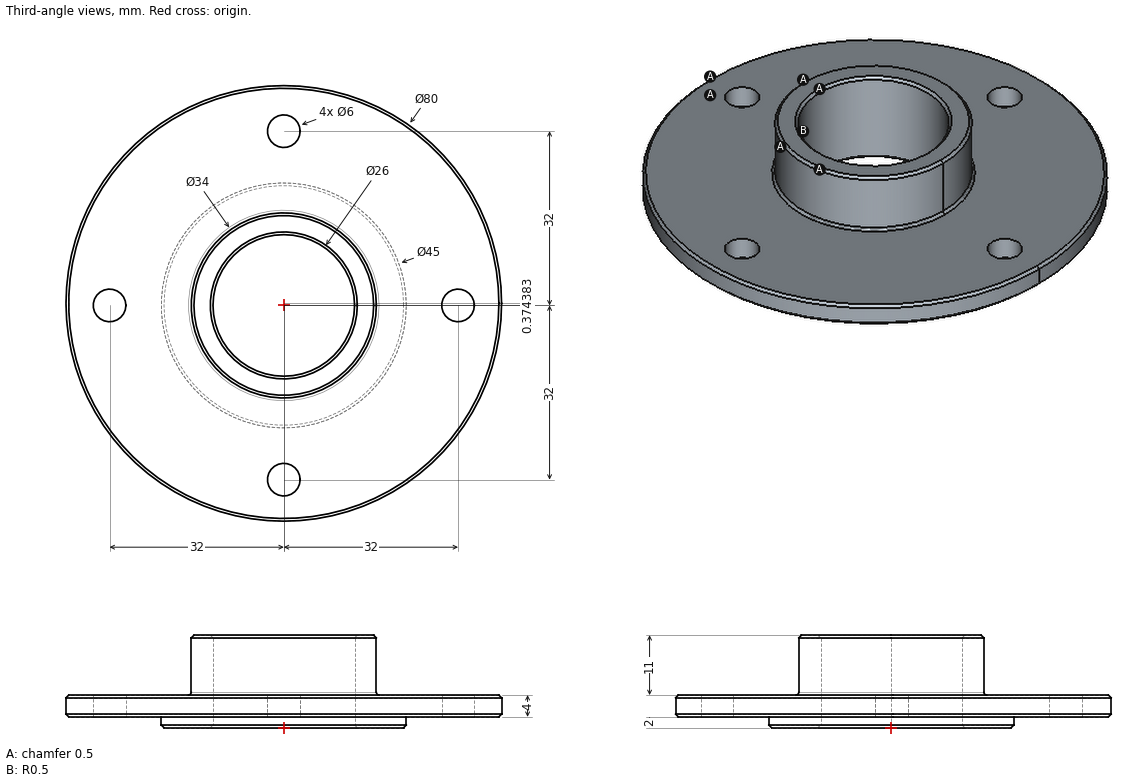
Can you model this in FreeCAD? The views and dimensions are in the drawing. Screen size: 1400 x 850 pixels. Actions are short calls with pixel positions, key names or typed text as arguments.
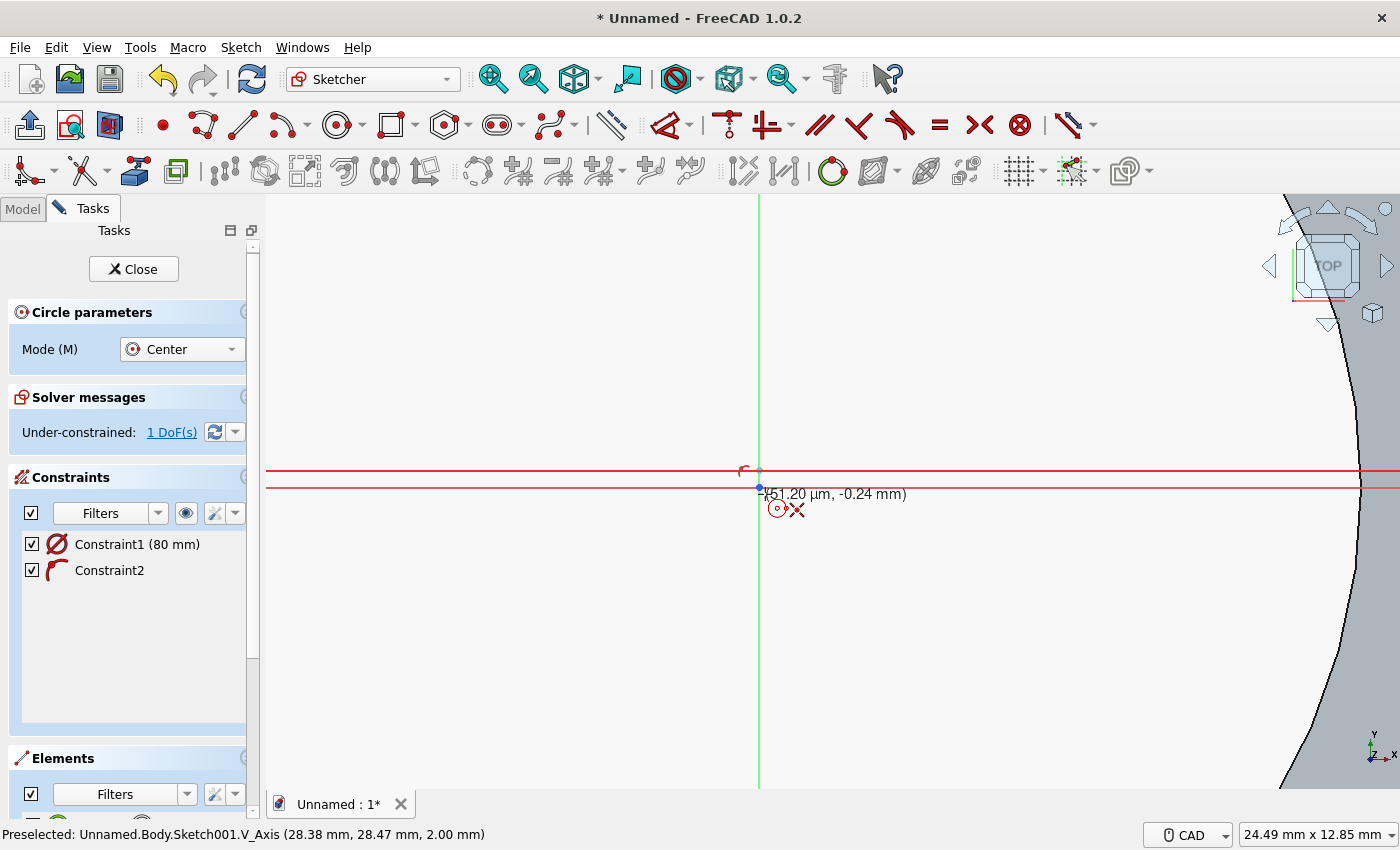
click(759, 488)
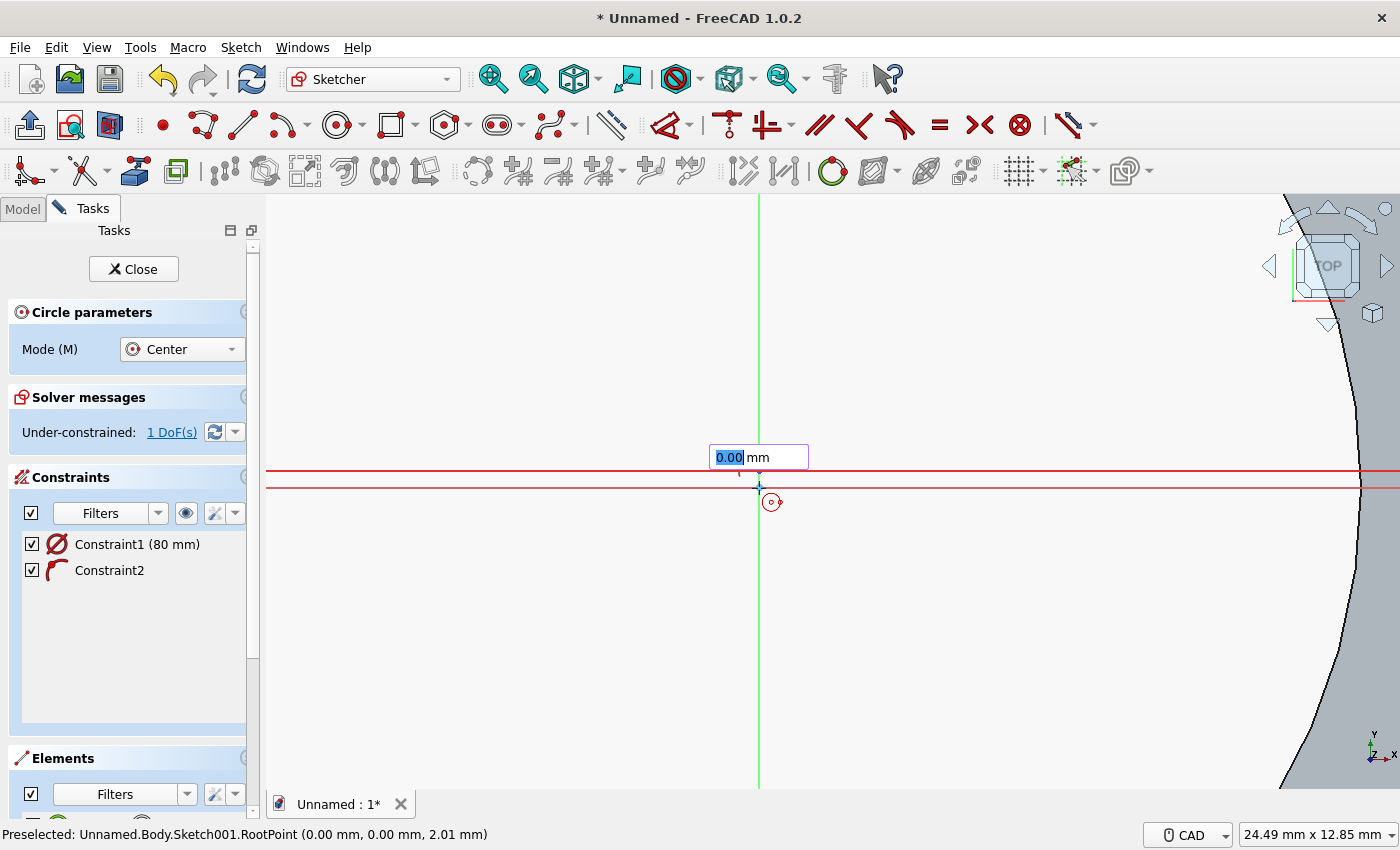
scroll(765, 494, down, 11)
move(812, 447)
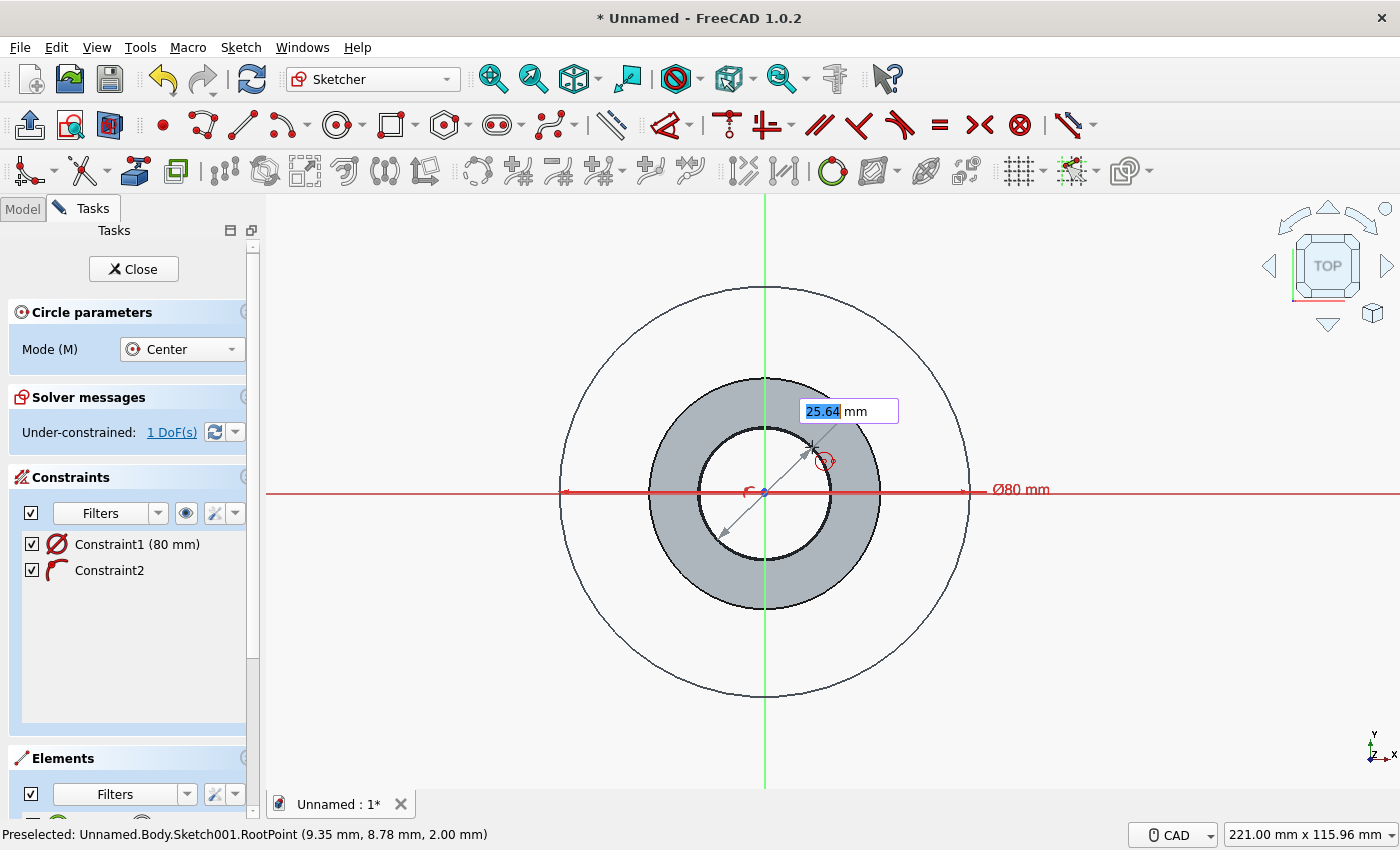
text(26)
key(Return)
key(Escape)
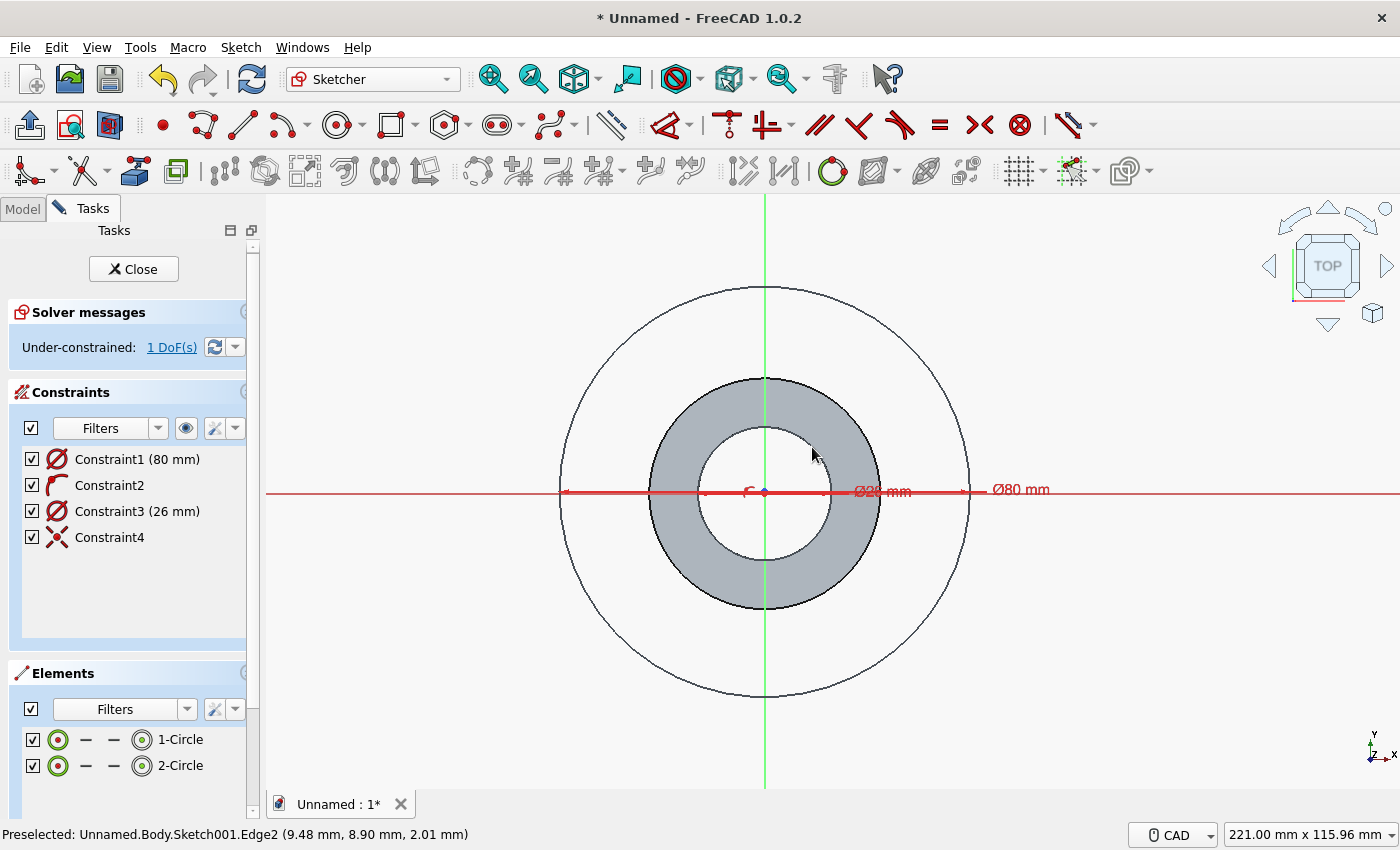
click(666, 126)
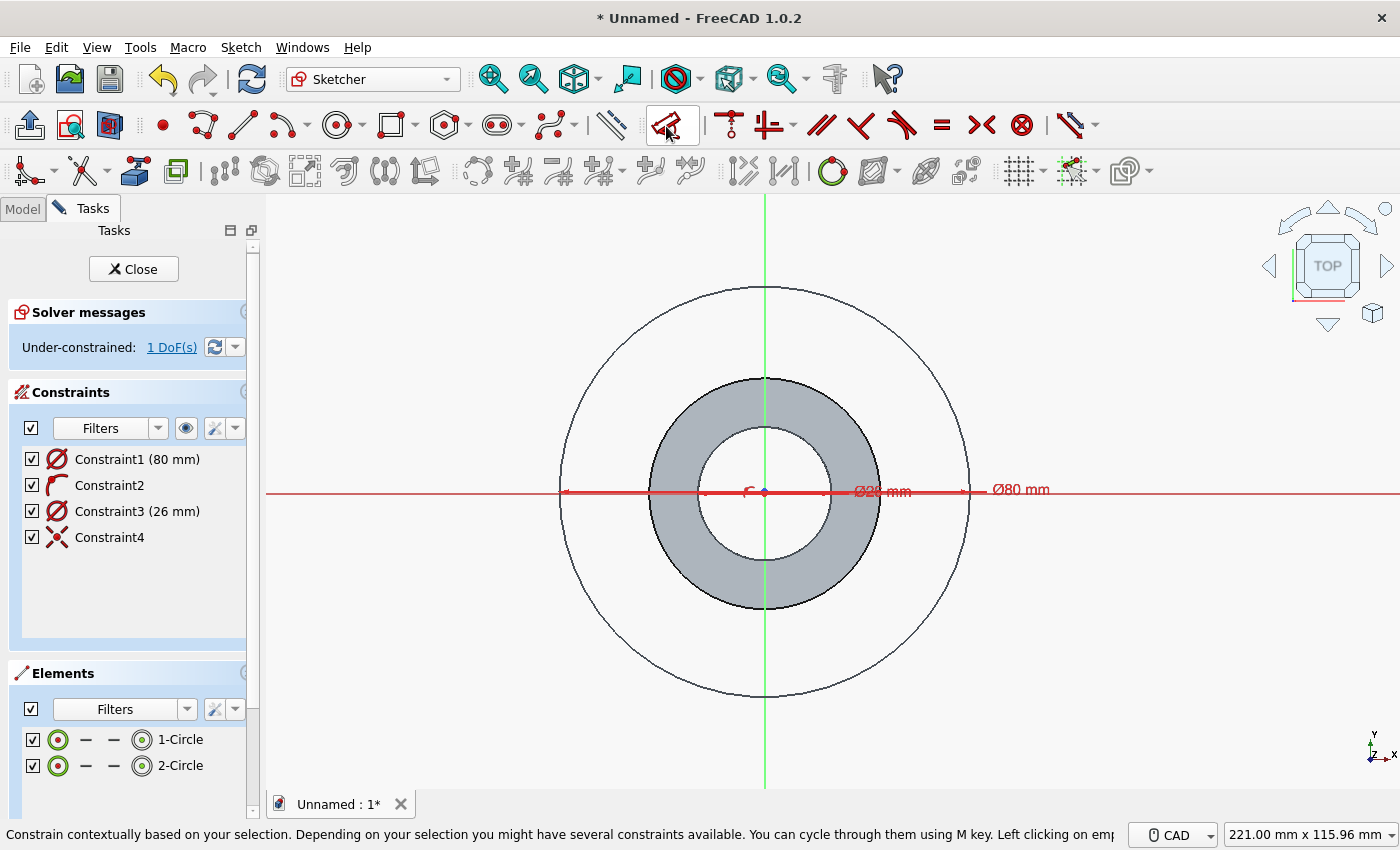
scroll(765, 492, up, 16)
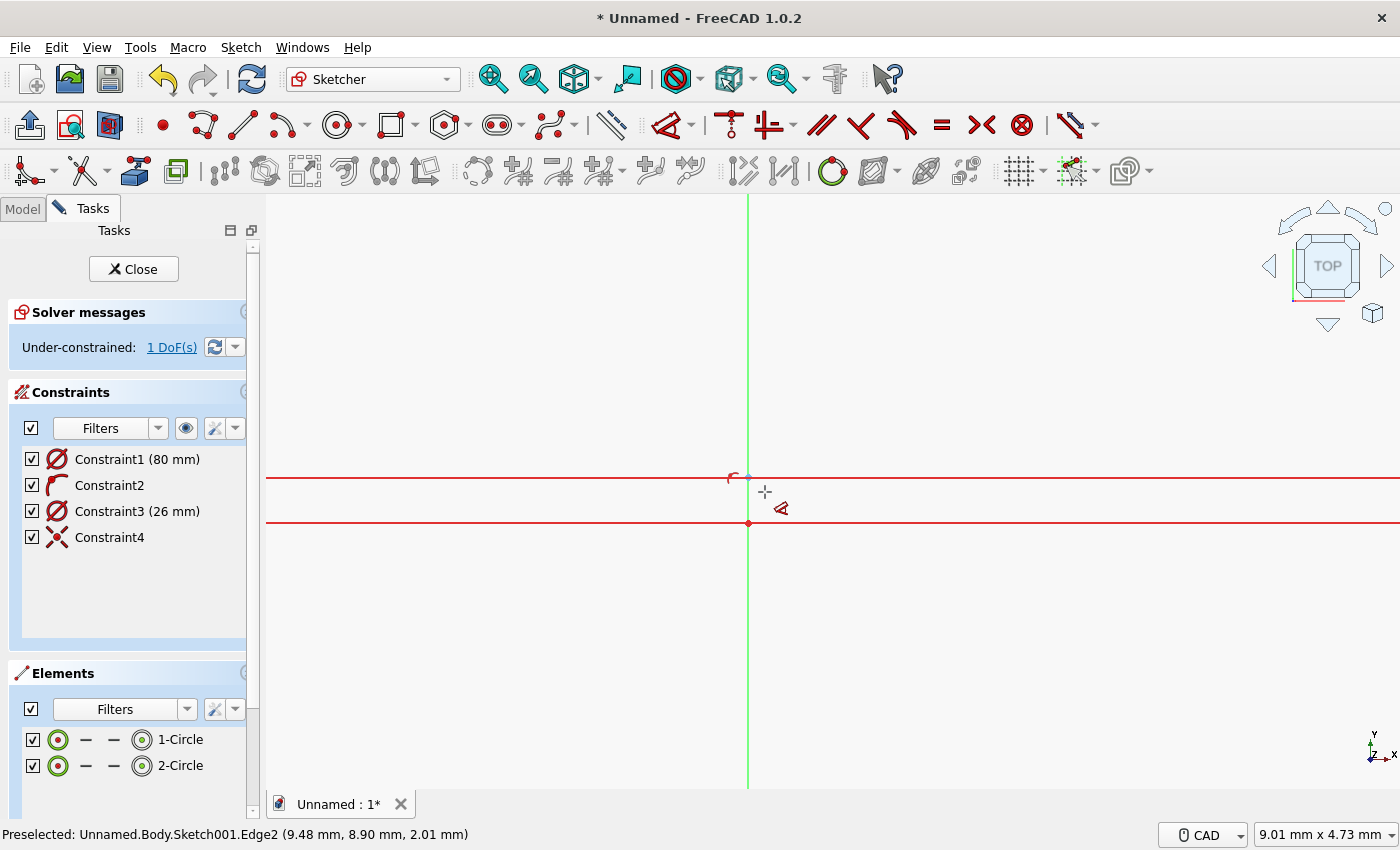
click(748, 478)
click(782, 500)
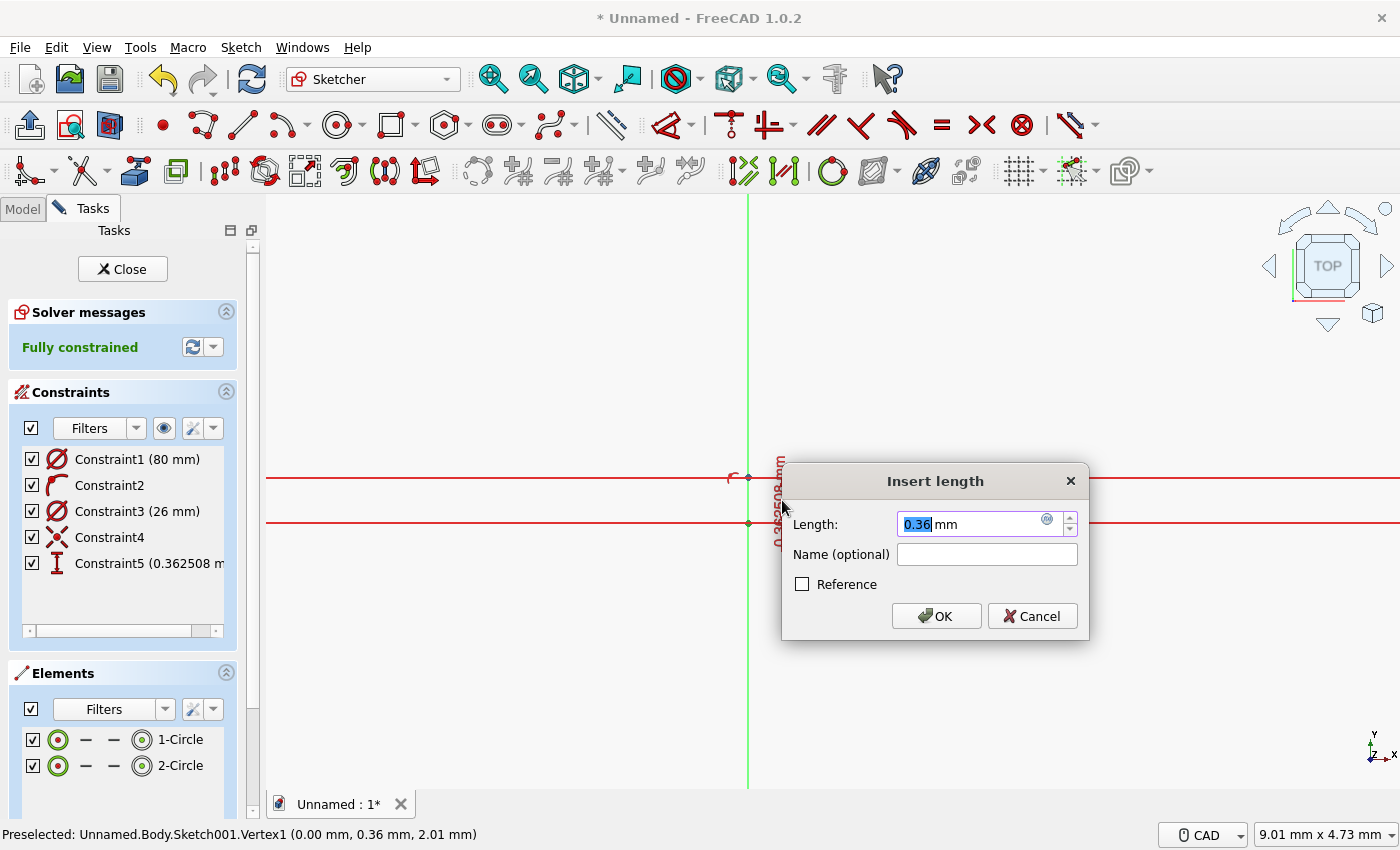
text(0.374383)
key(Return)
key(Escape)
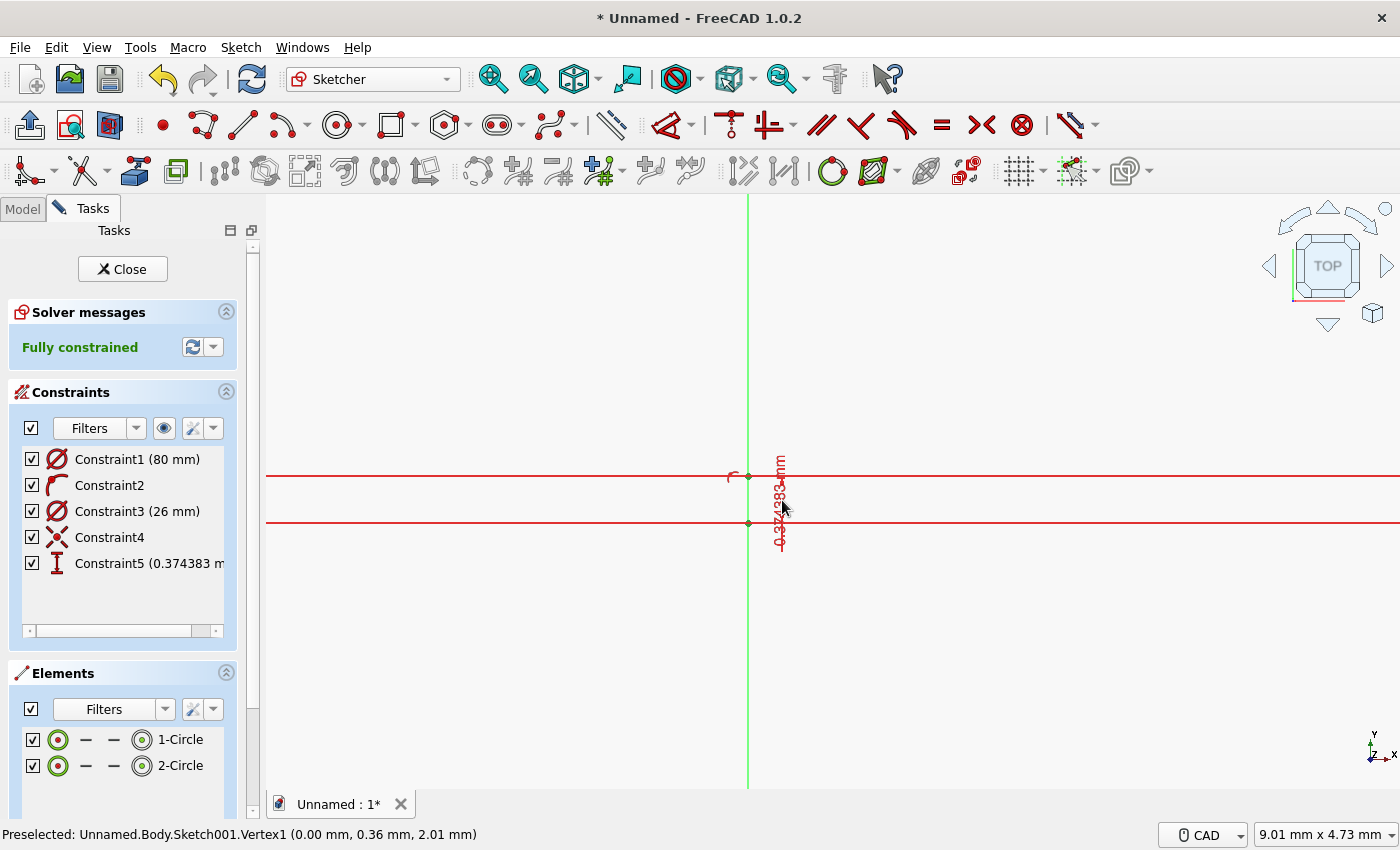
click(123, 269)